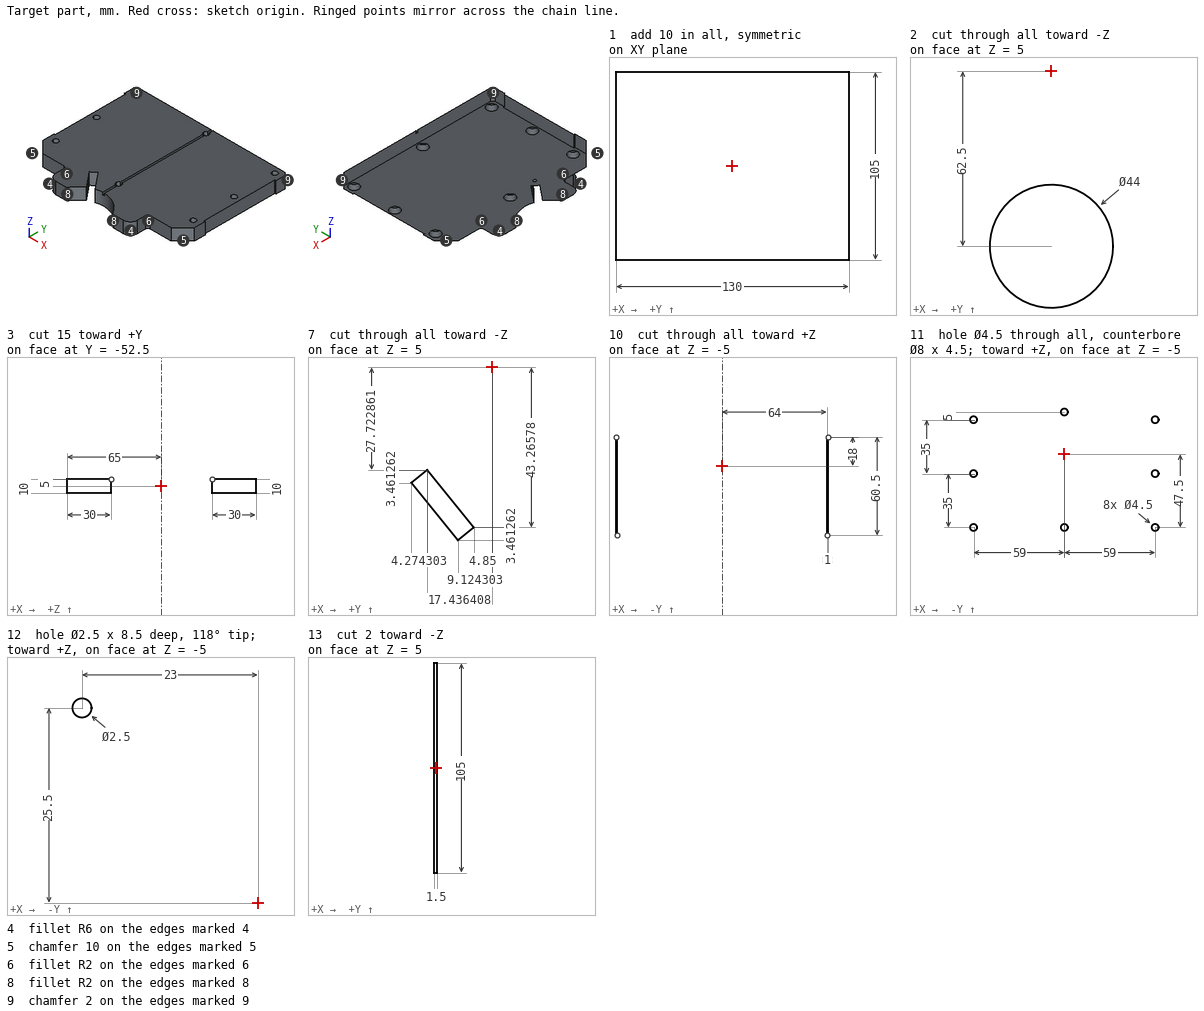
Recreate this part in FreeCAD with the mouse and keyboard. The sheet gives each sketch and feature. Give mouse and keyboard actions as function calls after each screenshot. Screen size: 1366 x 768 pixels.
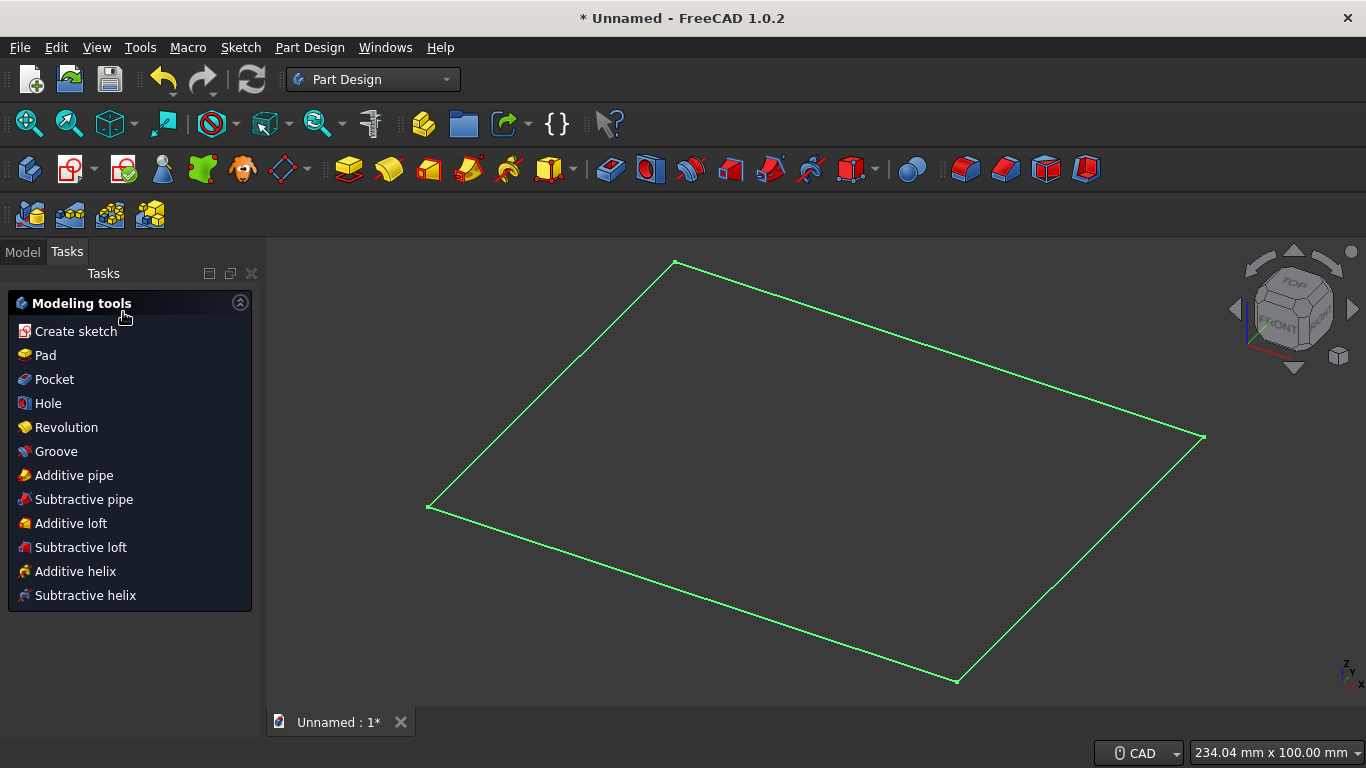
click(350, 170)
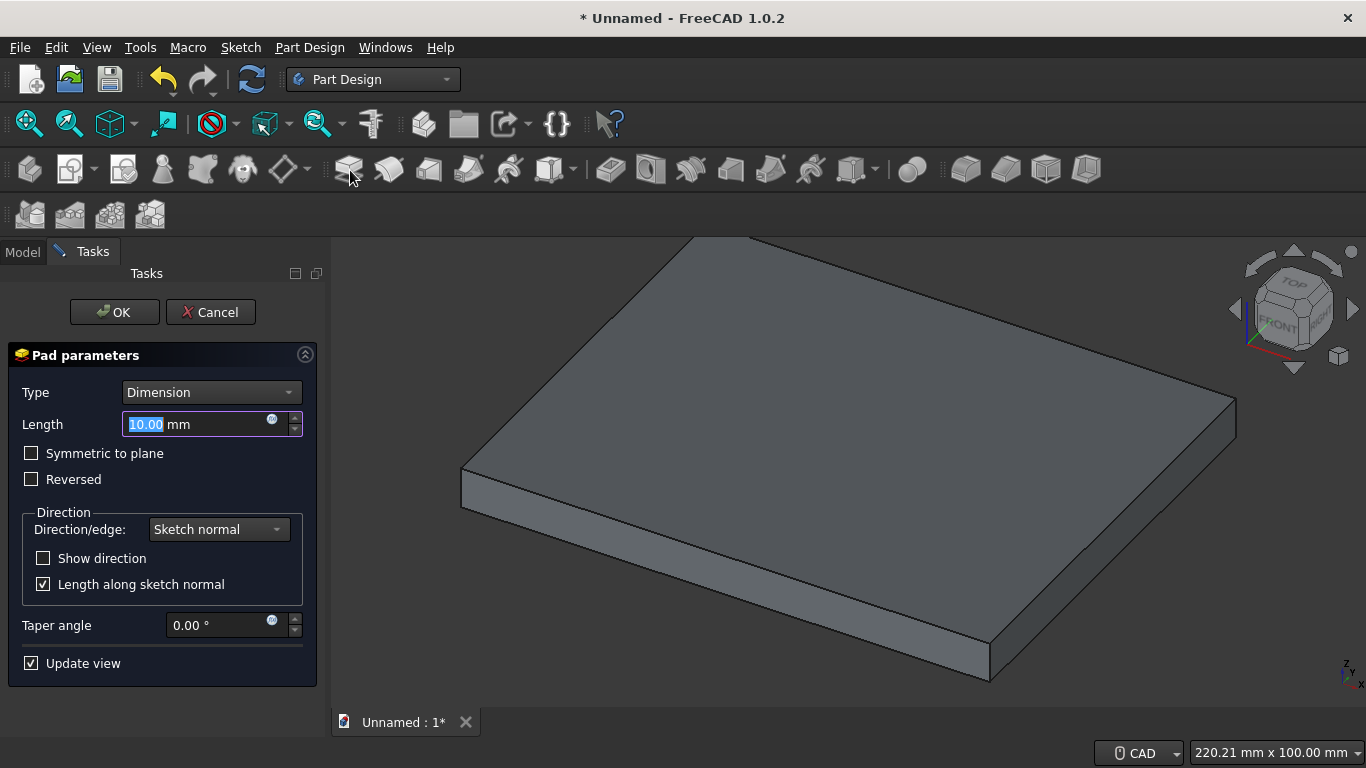
text(10)
key(Tab)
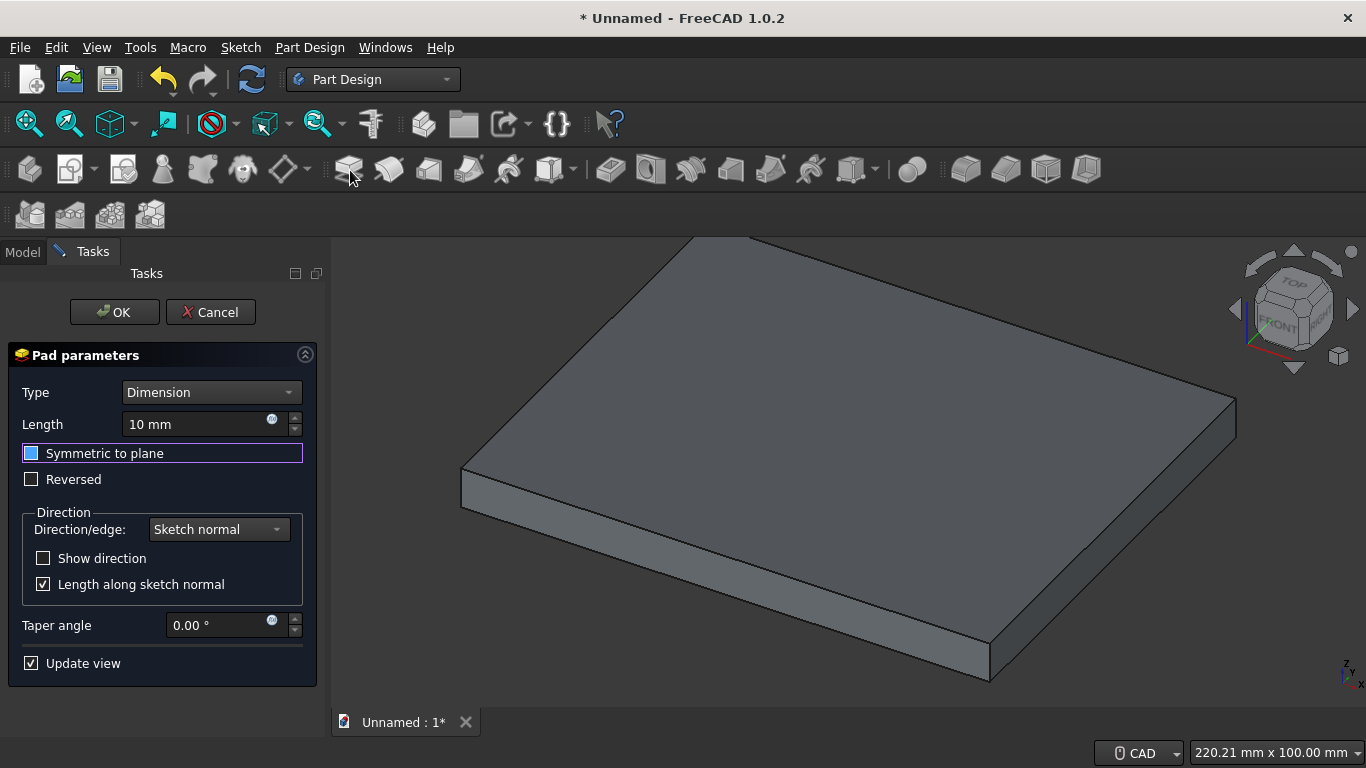
click(30, 453)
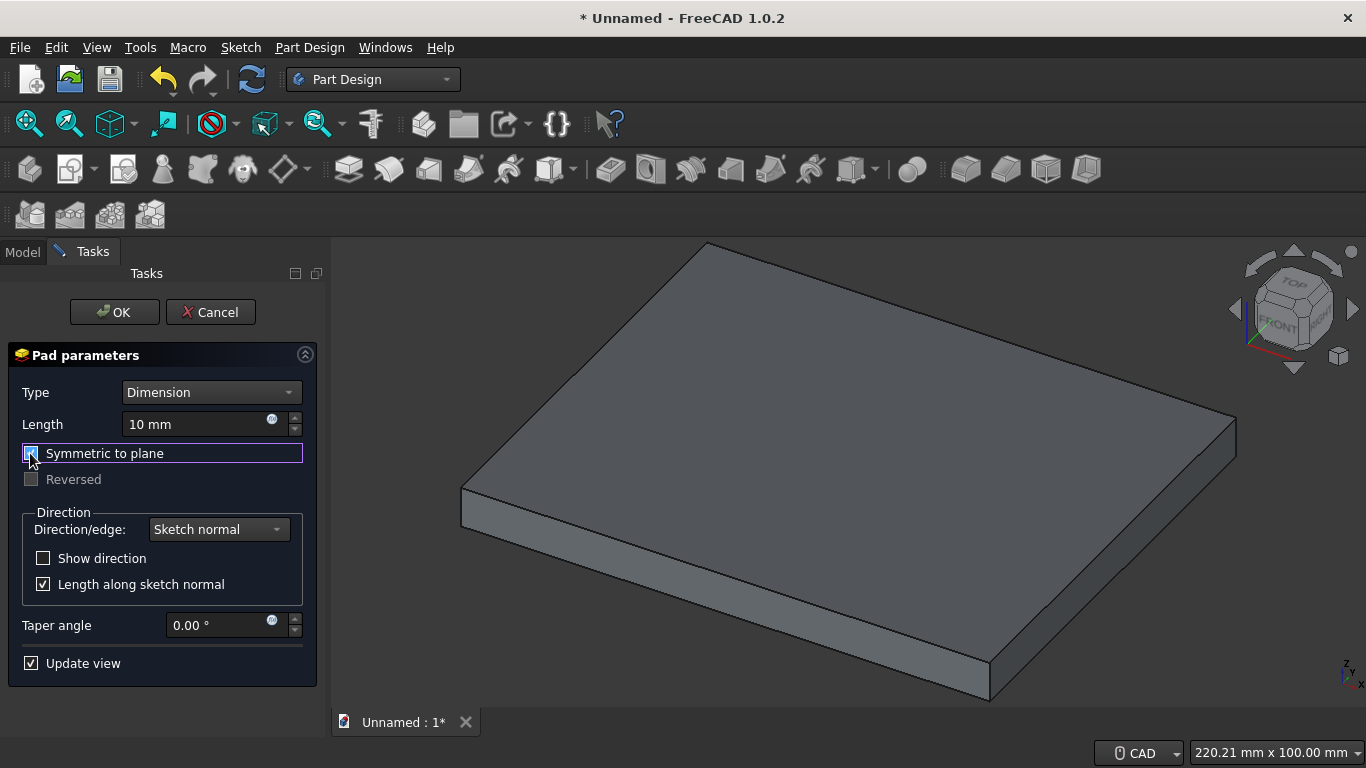
click(115, 312)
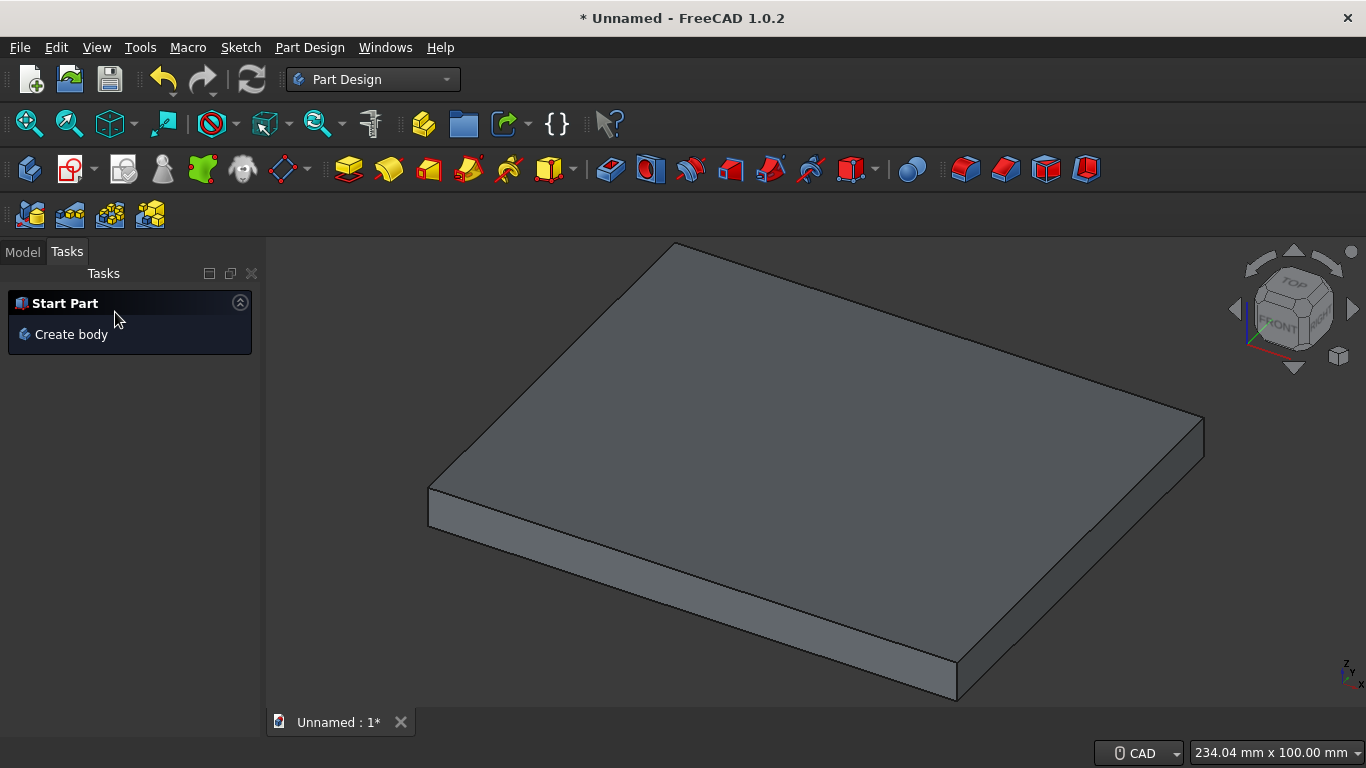
click(816, 452)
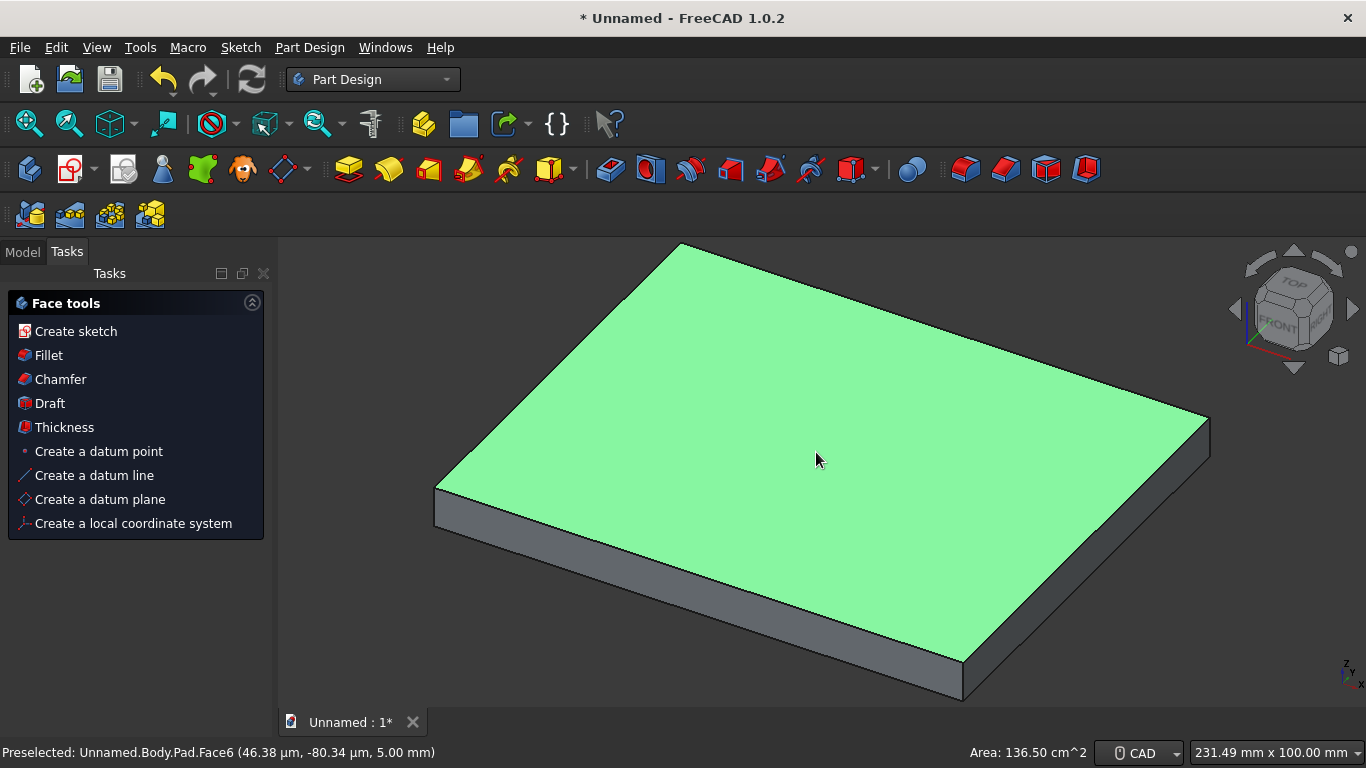
click(70, 170)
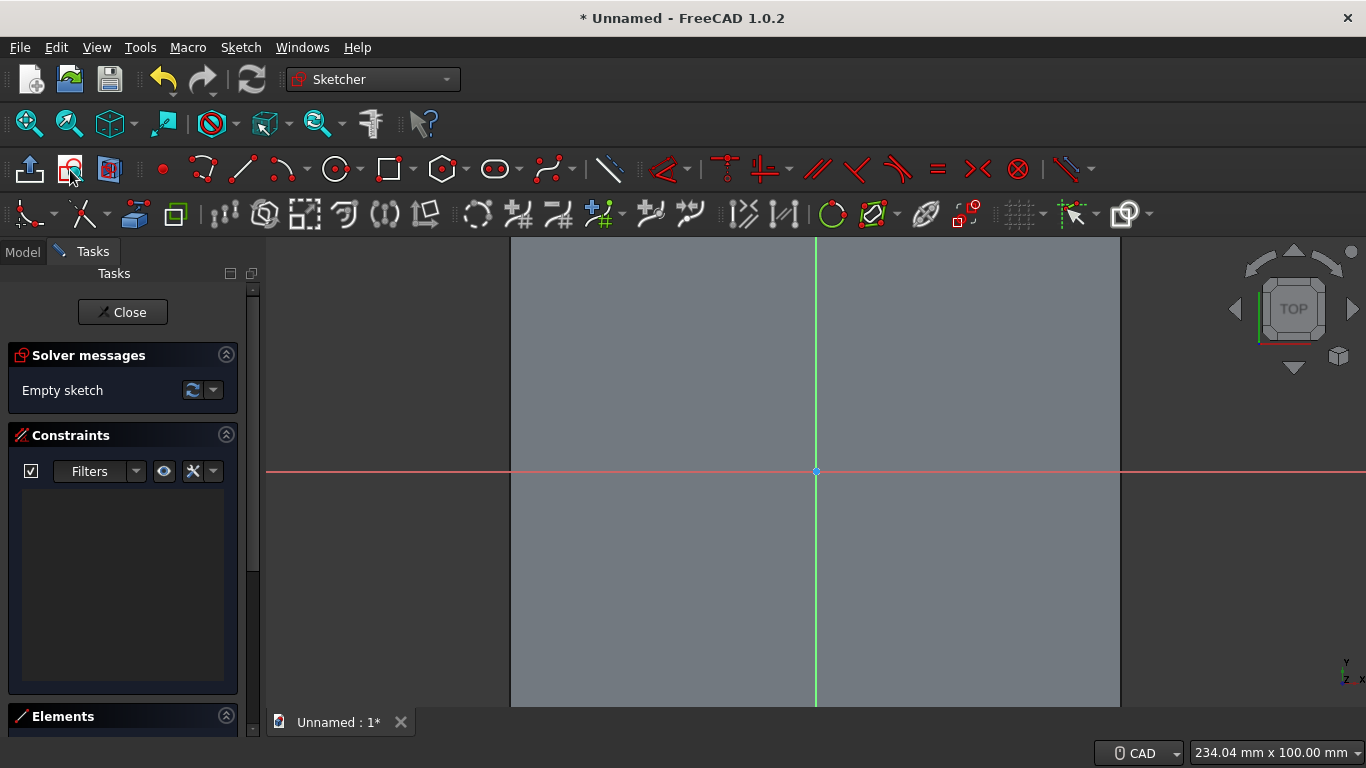
scroll(664, 265, down, 3)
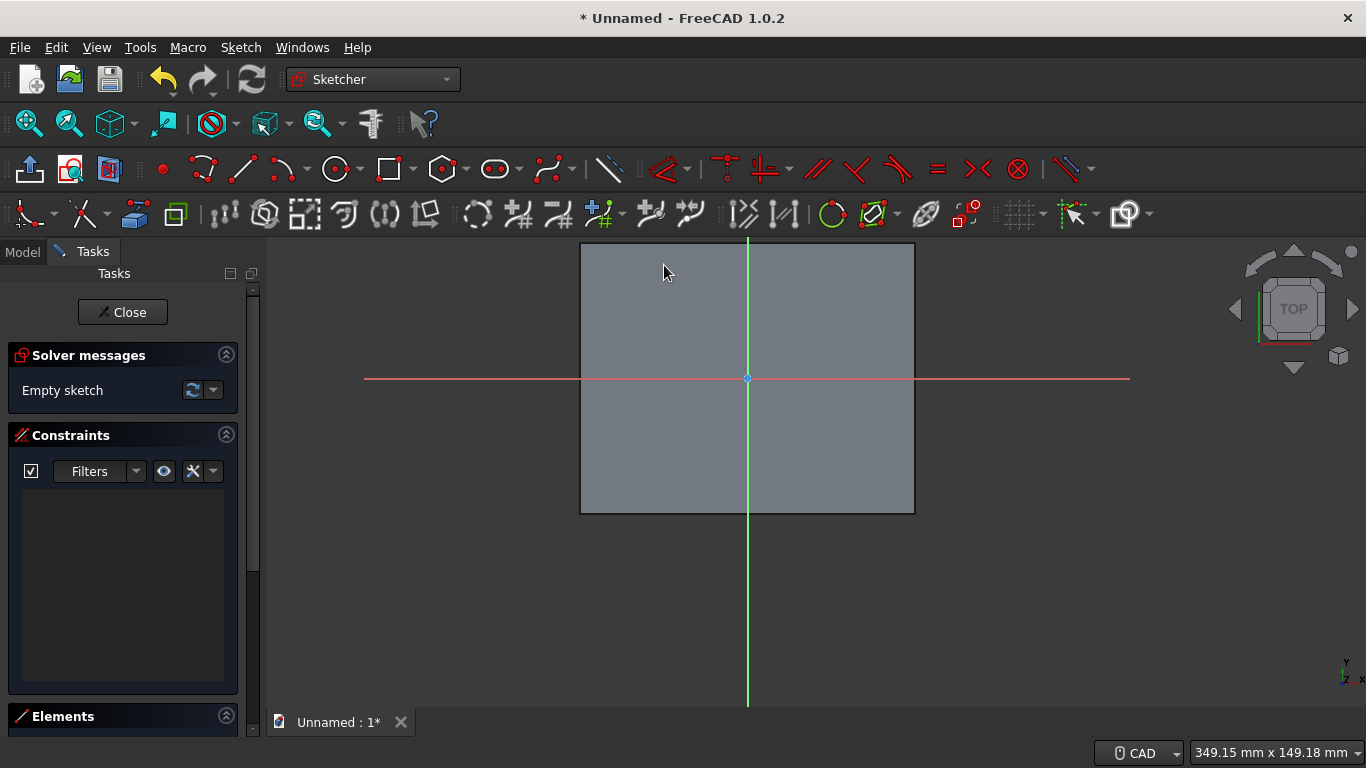
click(336, 170)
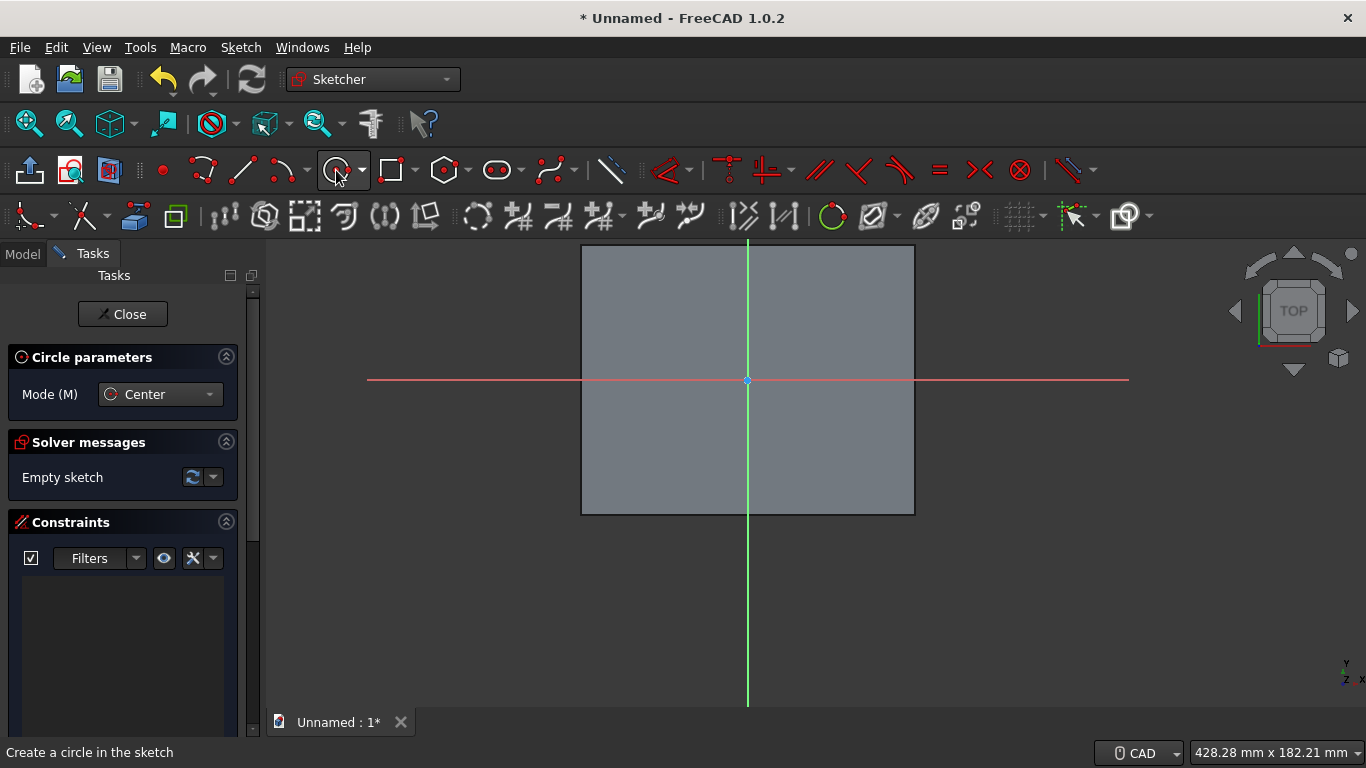
click(748, 541)
move(788, 501)